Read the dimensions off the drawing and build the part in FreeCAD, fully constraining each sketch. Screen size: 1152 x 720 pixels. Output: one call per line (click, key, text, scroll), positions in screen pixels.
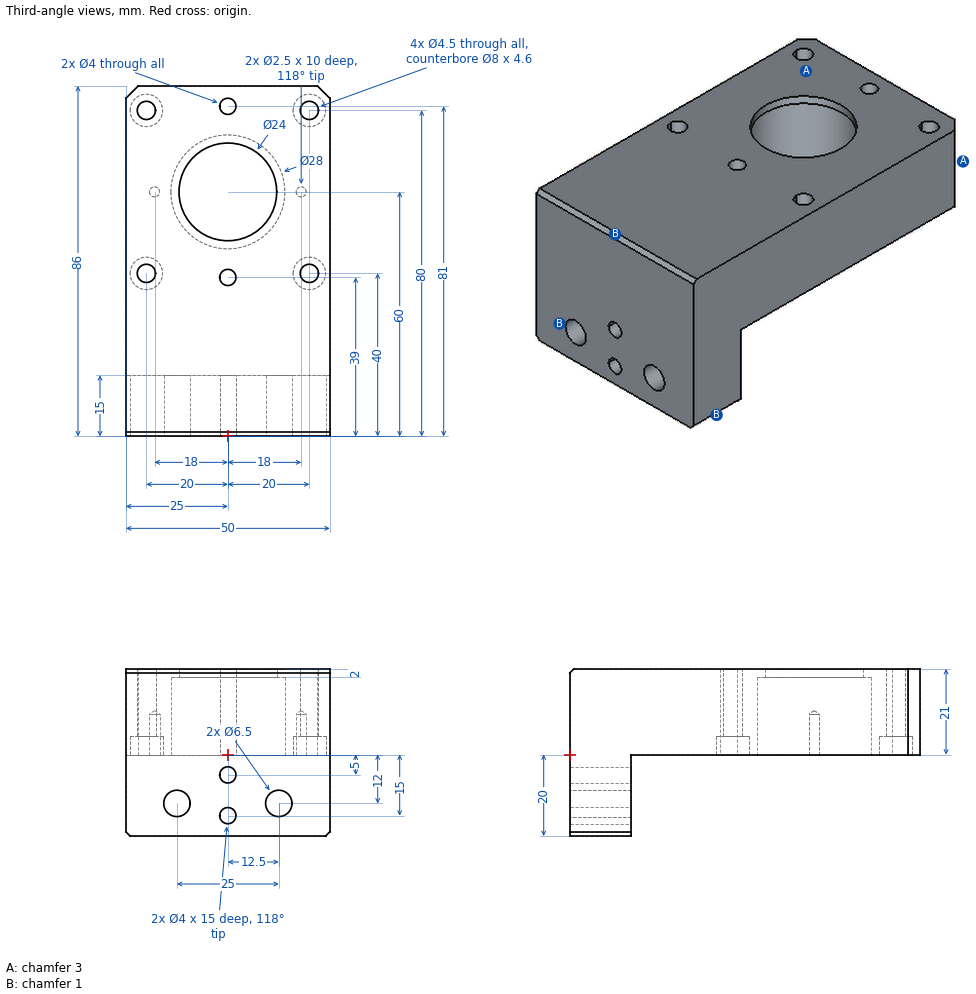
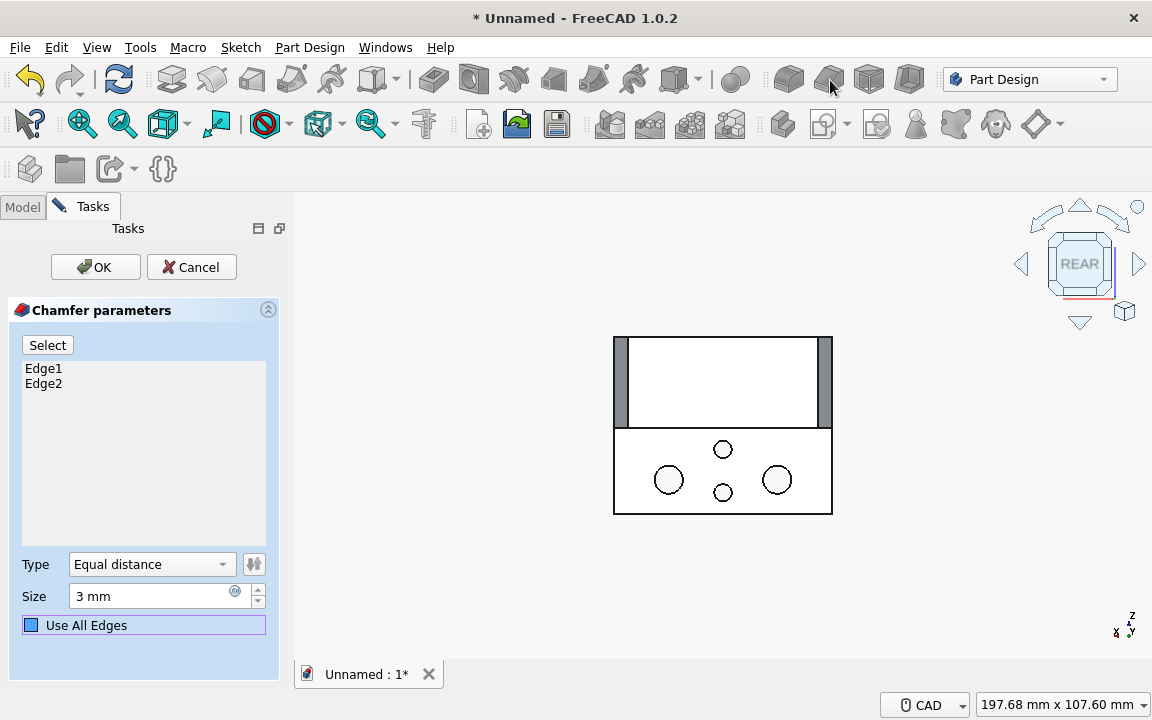
click(96, 267)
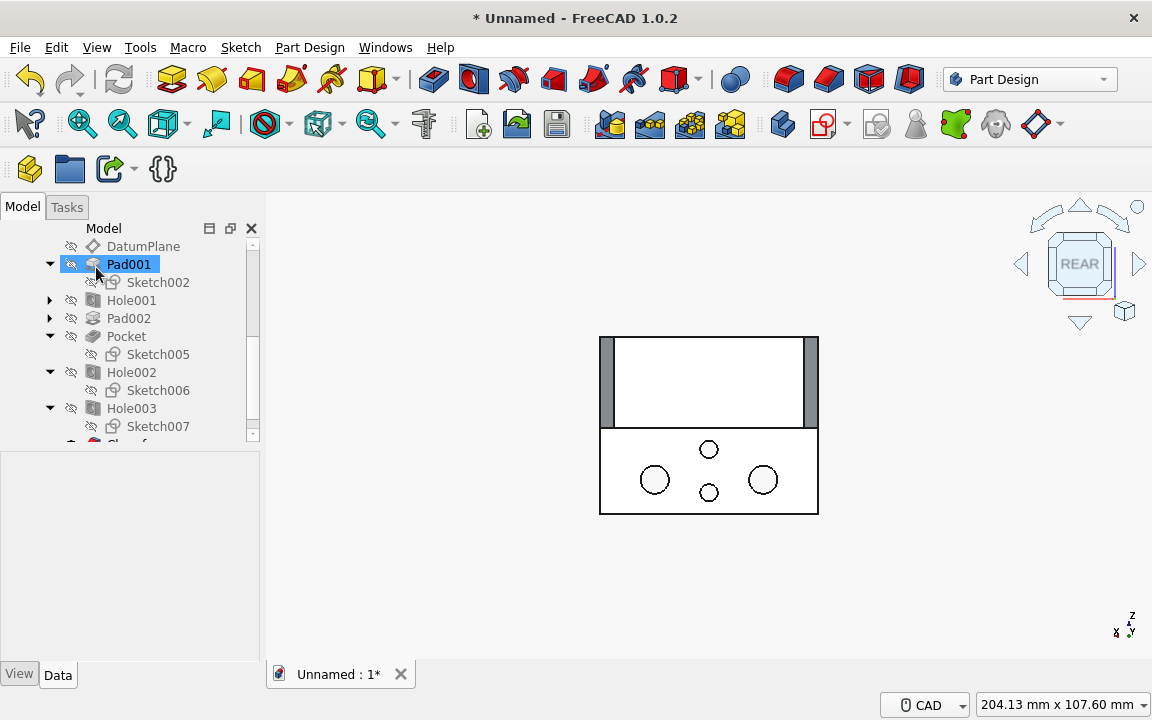
click(84, 124)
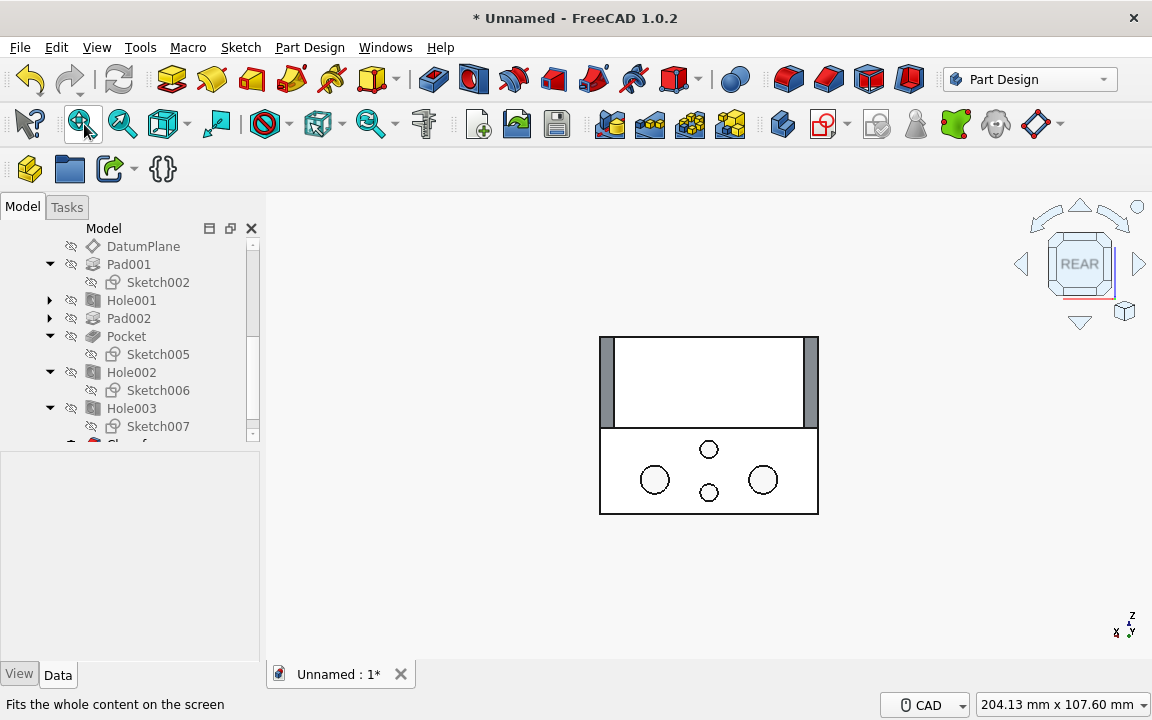
key(0)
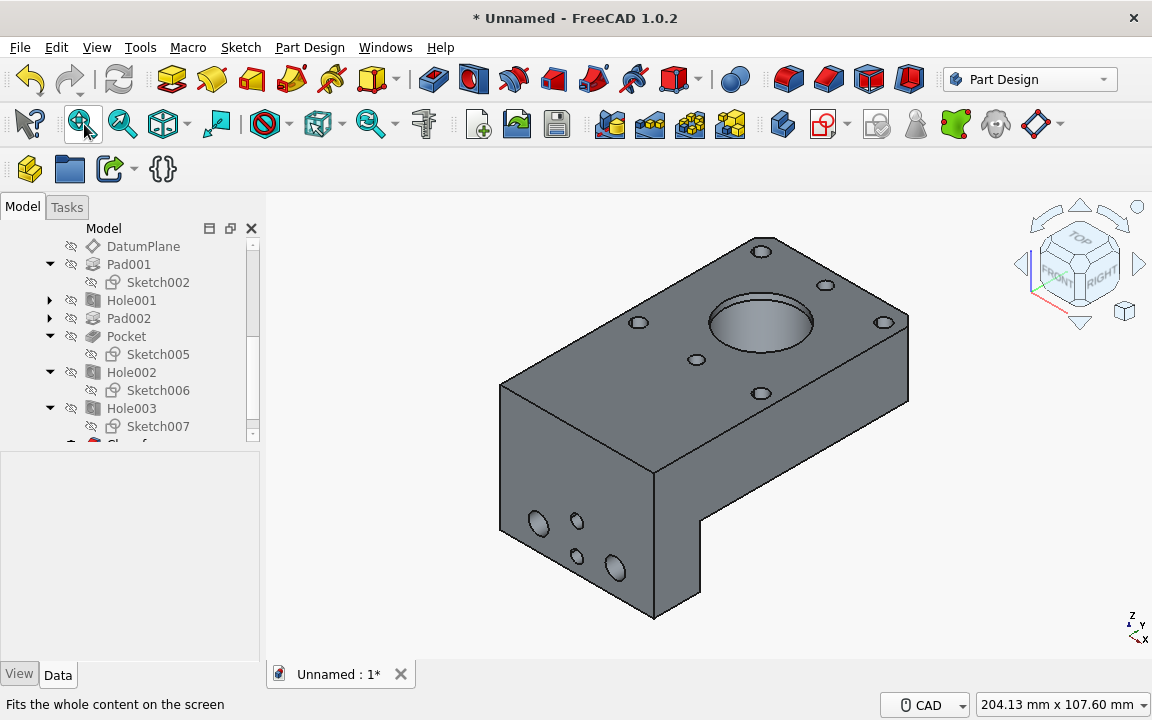
click(577, 428)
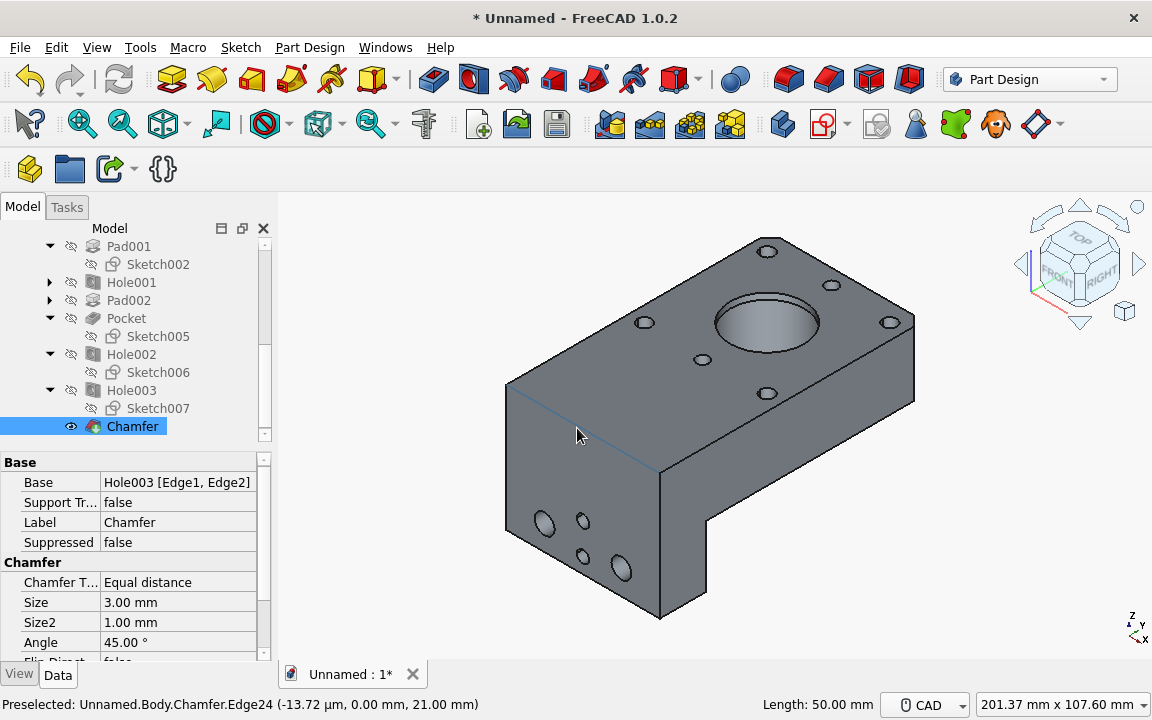
key(2)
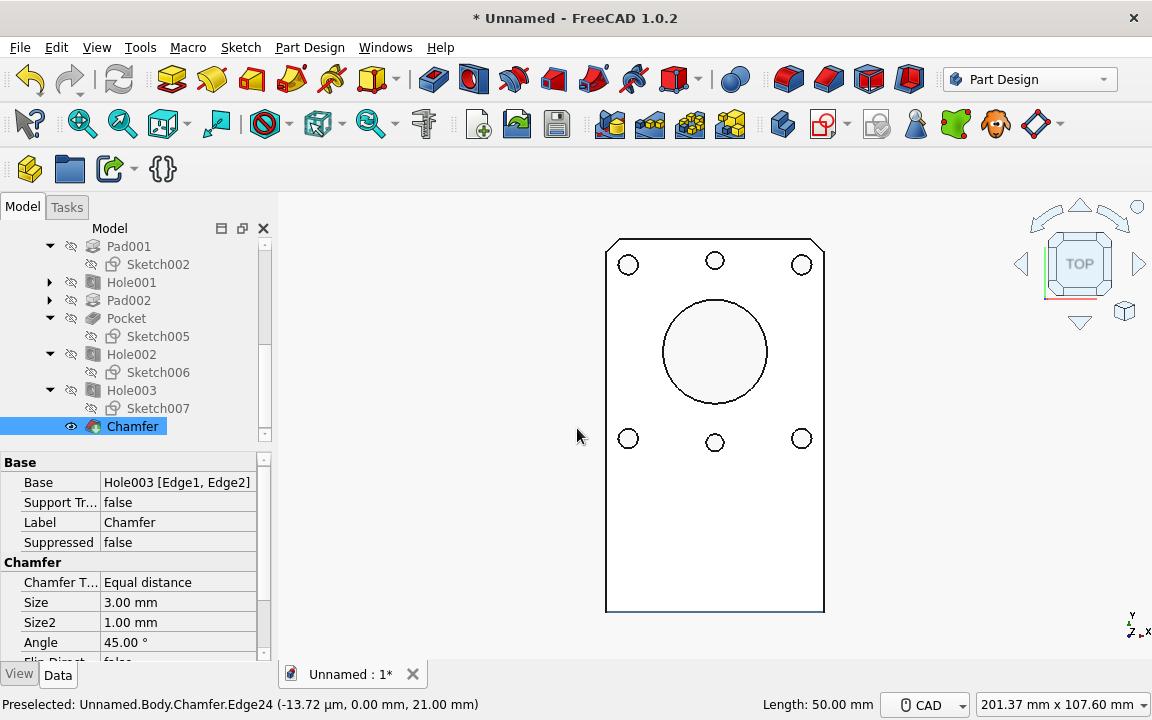
key(1)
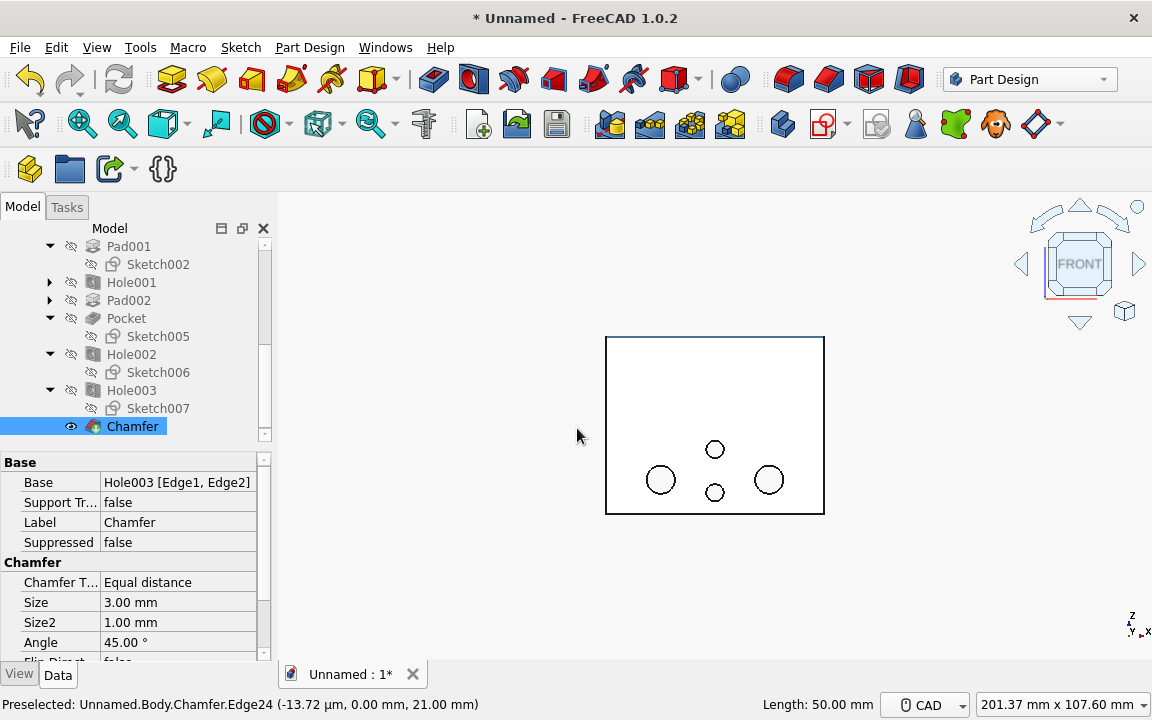
click(84, 124)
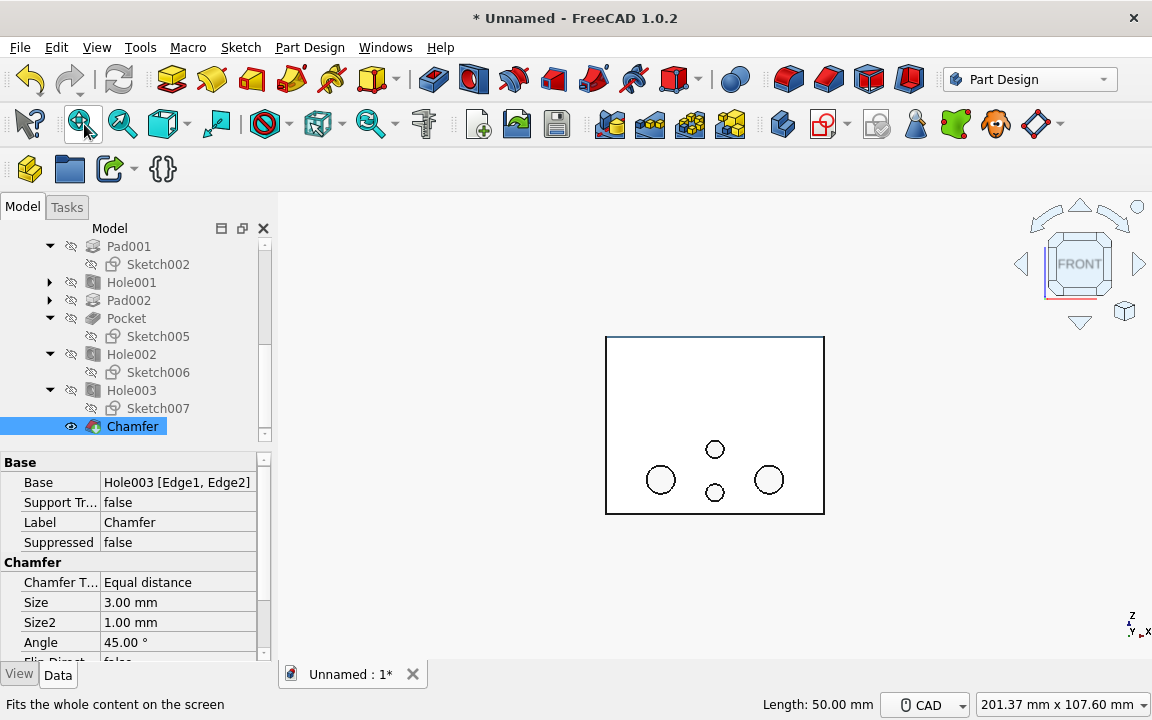
key(3)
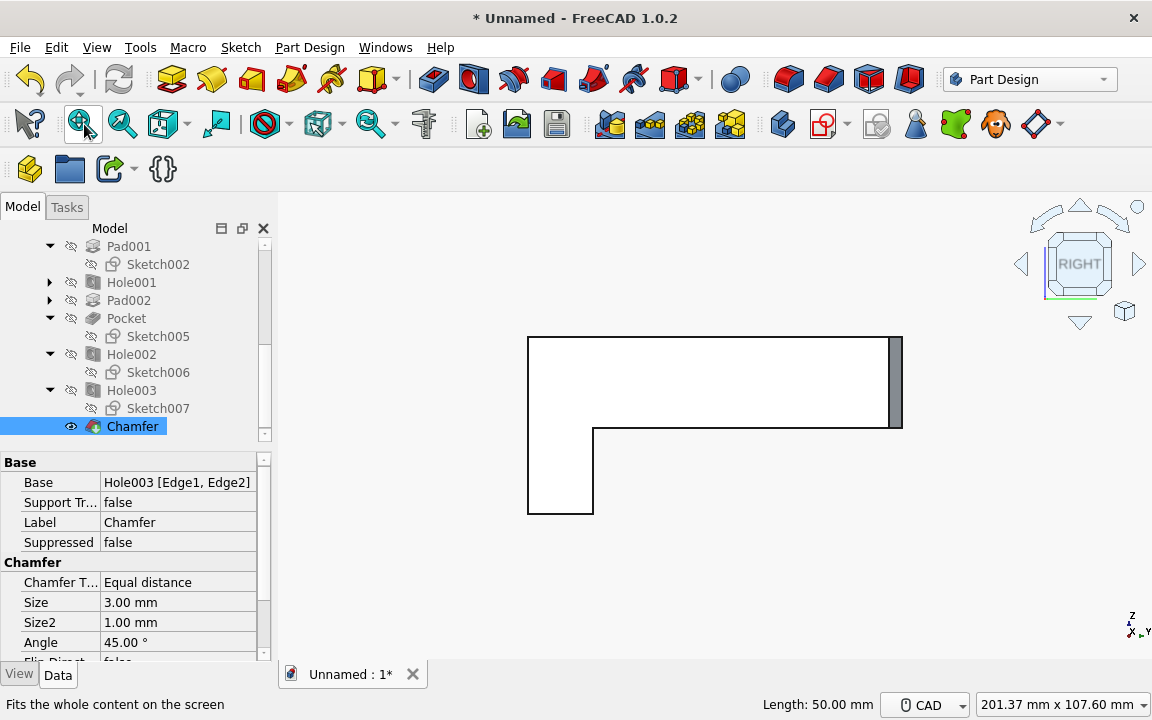
key(v)
key(f)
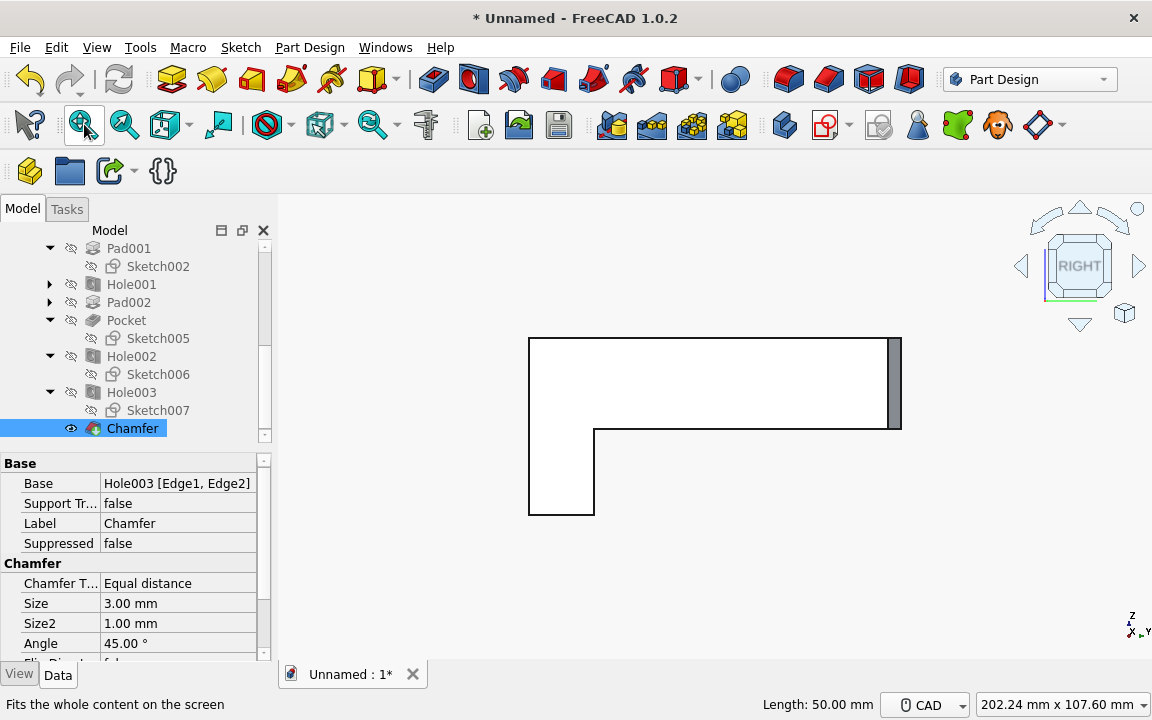
click(562, 514, ctrl)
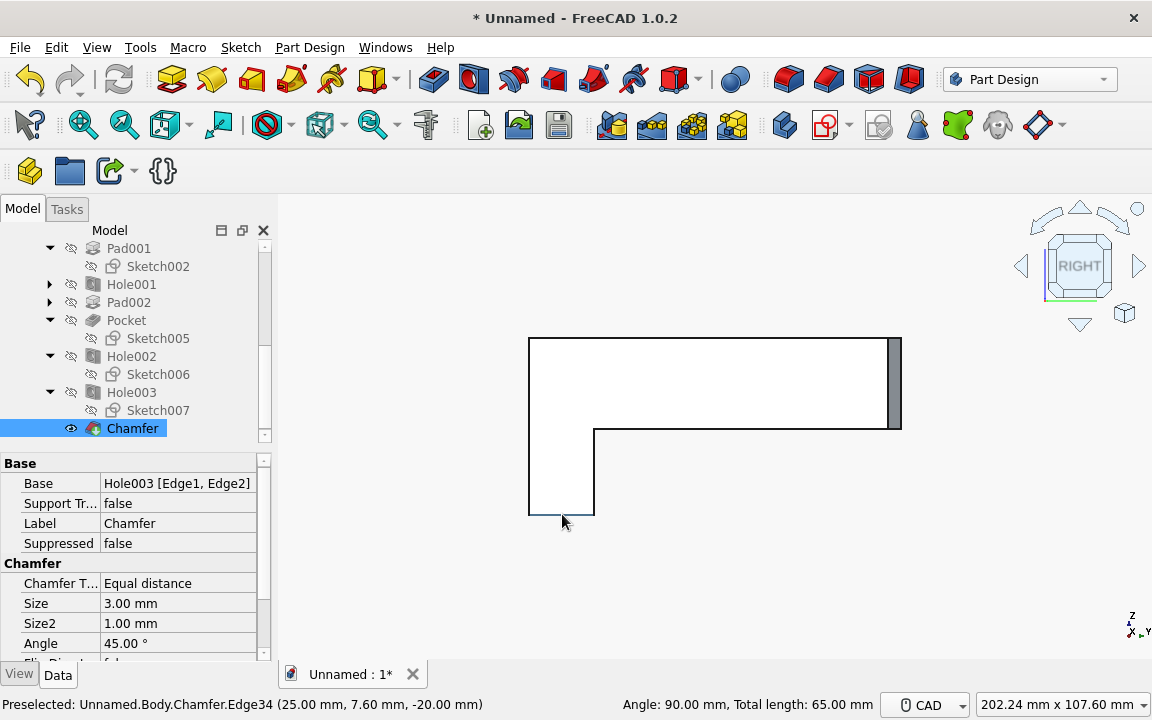
key(5)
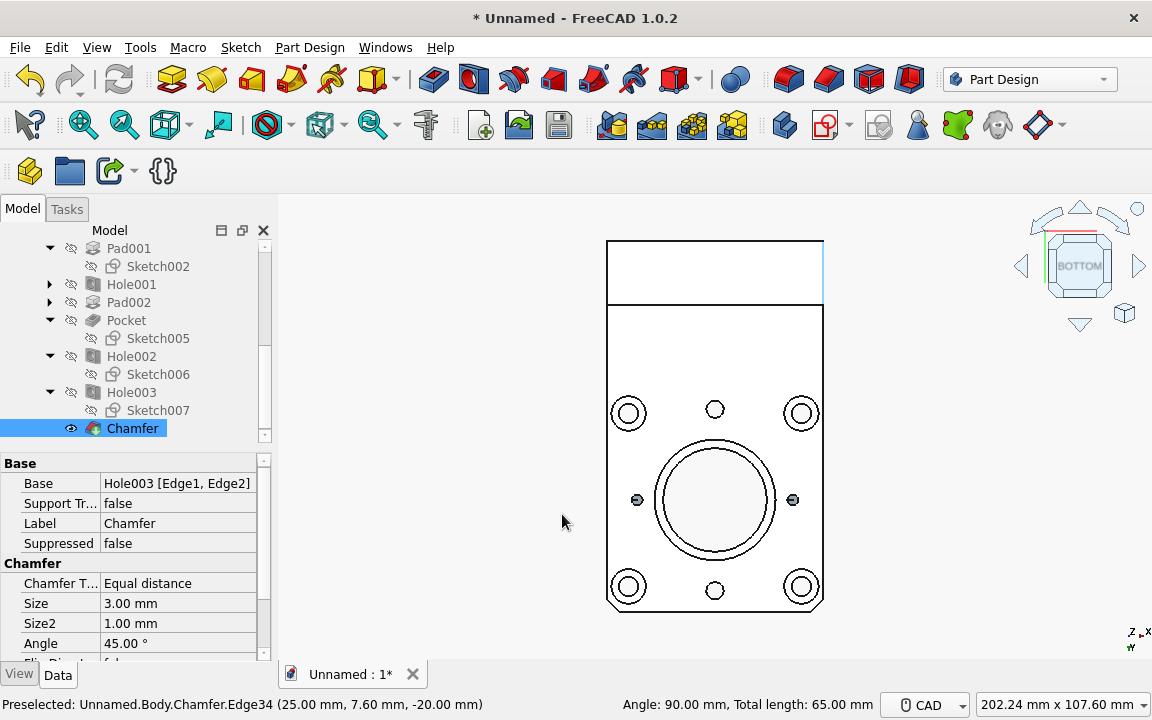
click(607, 272, ctrl)